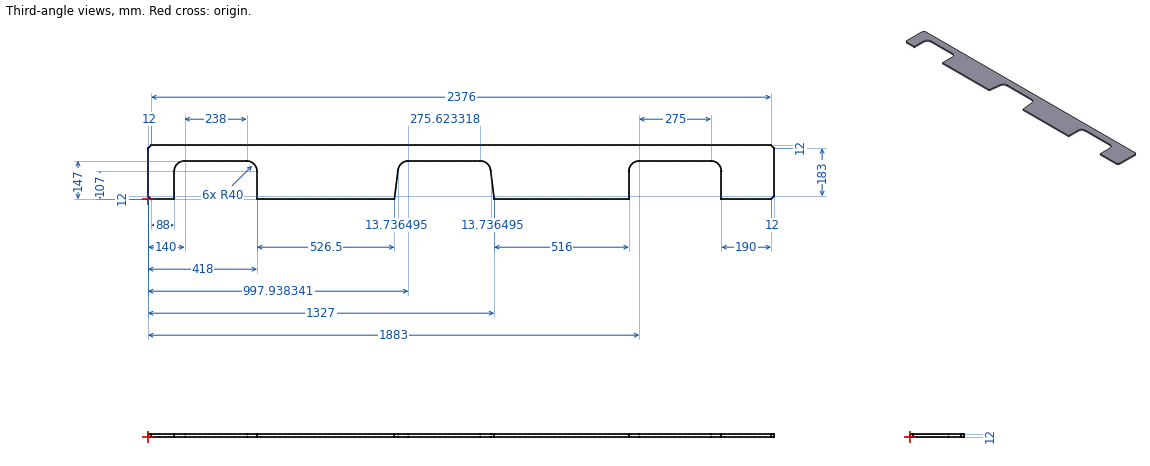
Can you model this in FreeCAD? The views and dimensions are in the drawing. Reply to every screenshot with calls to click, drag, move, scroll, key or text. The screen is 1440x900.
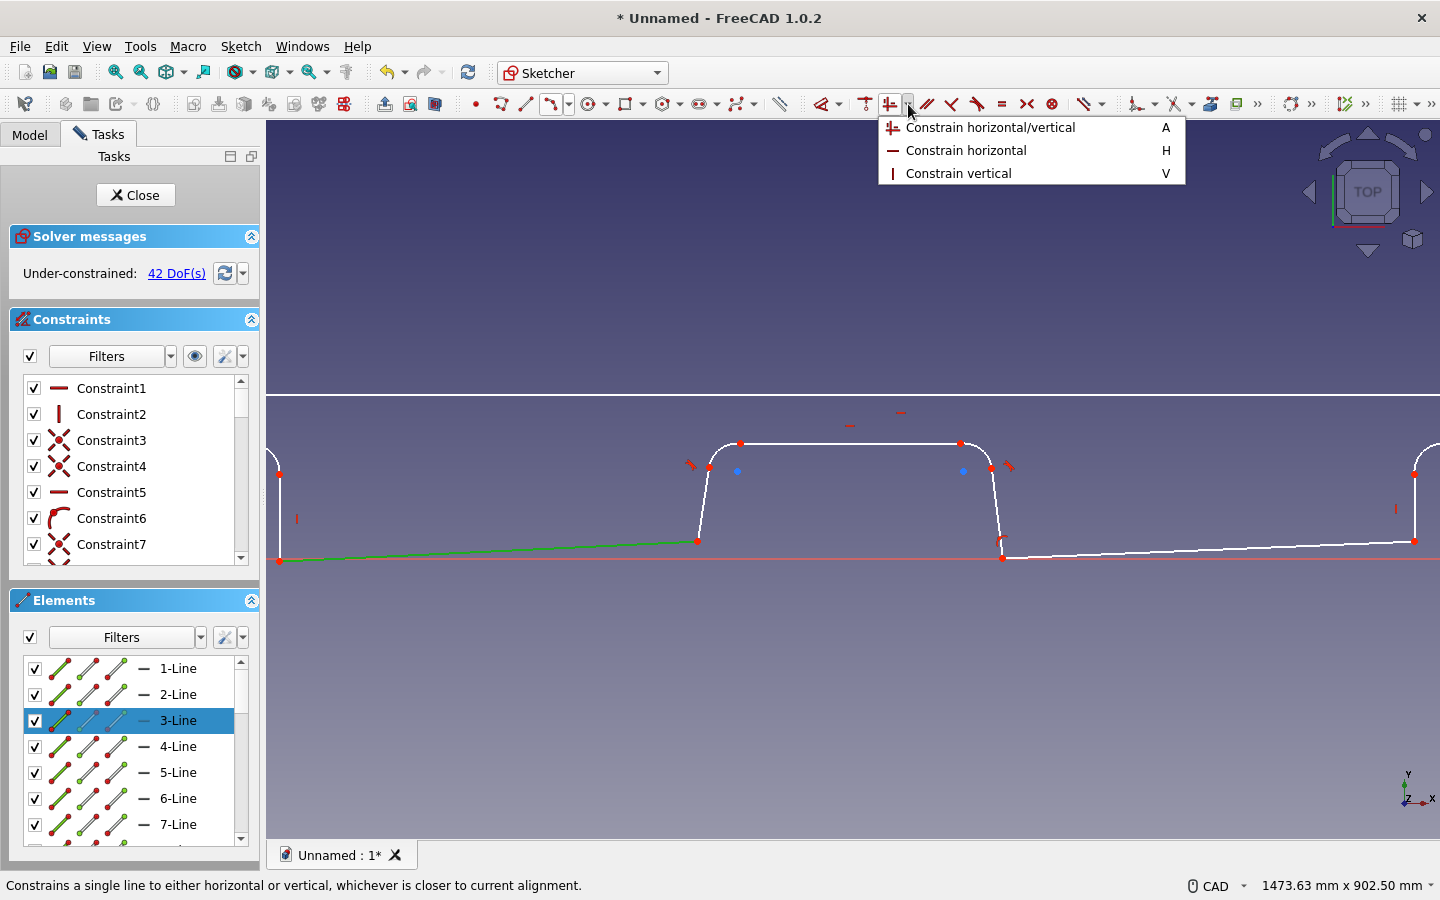
click(1032, 150)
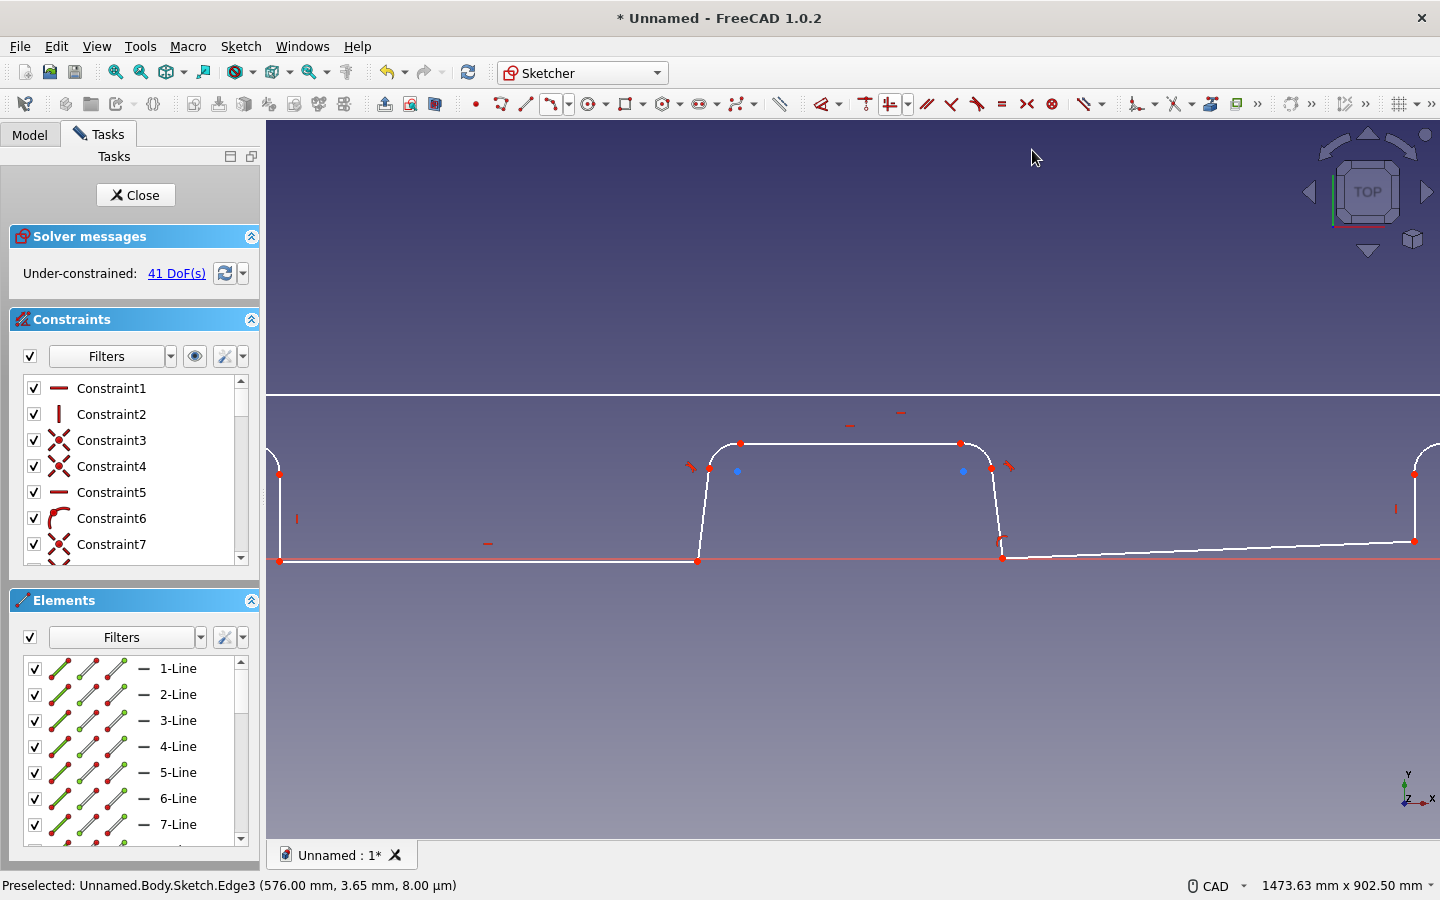
scroll(1250, 548, up, 2)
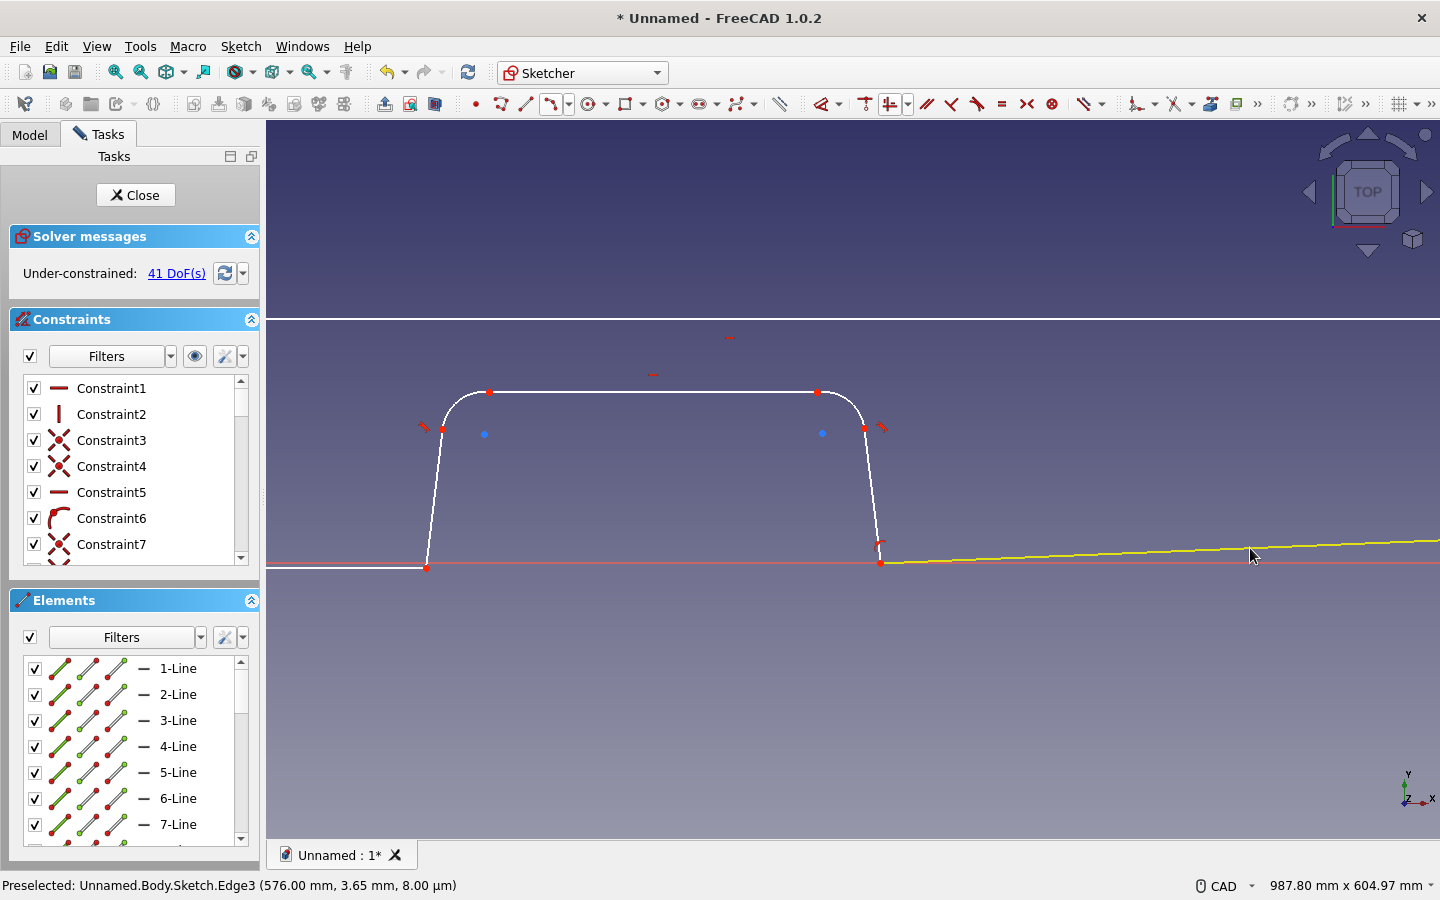
click(1249, 548)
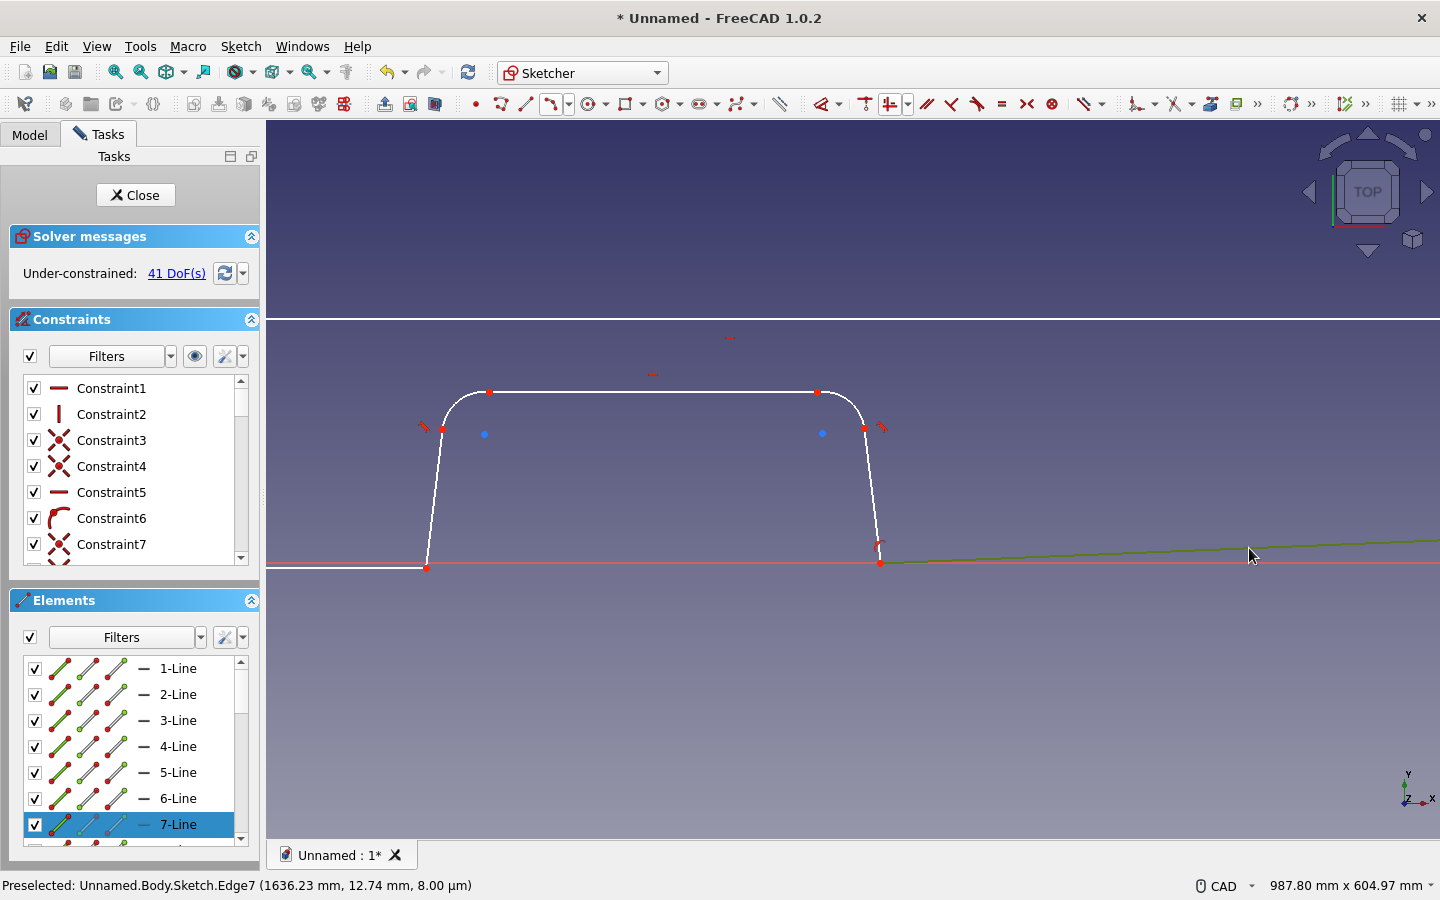
click(908, 104)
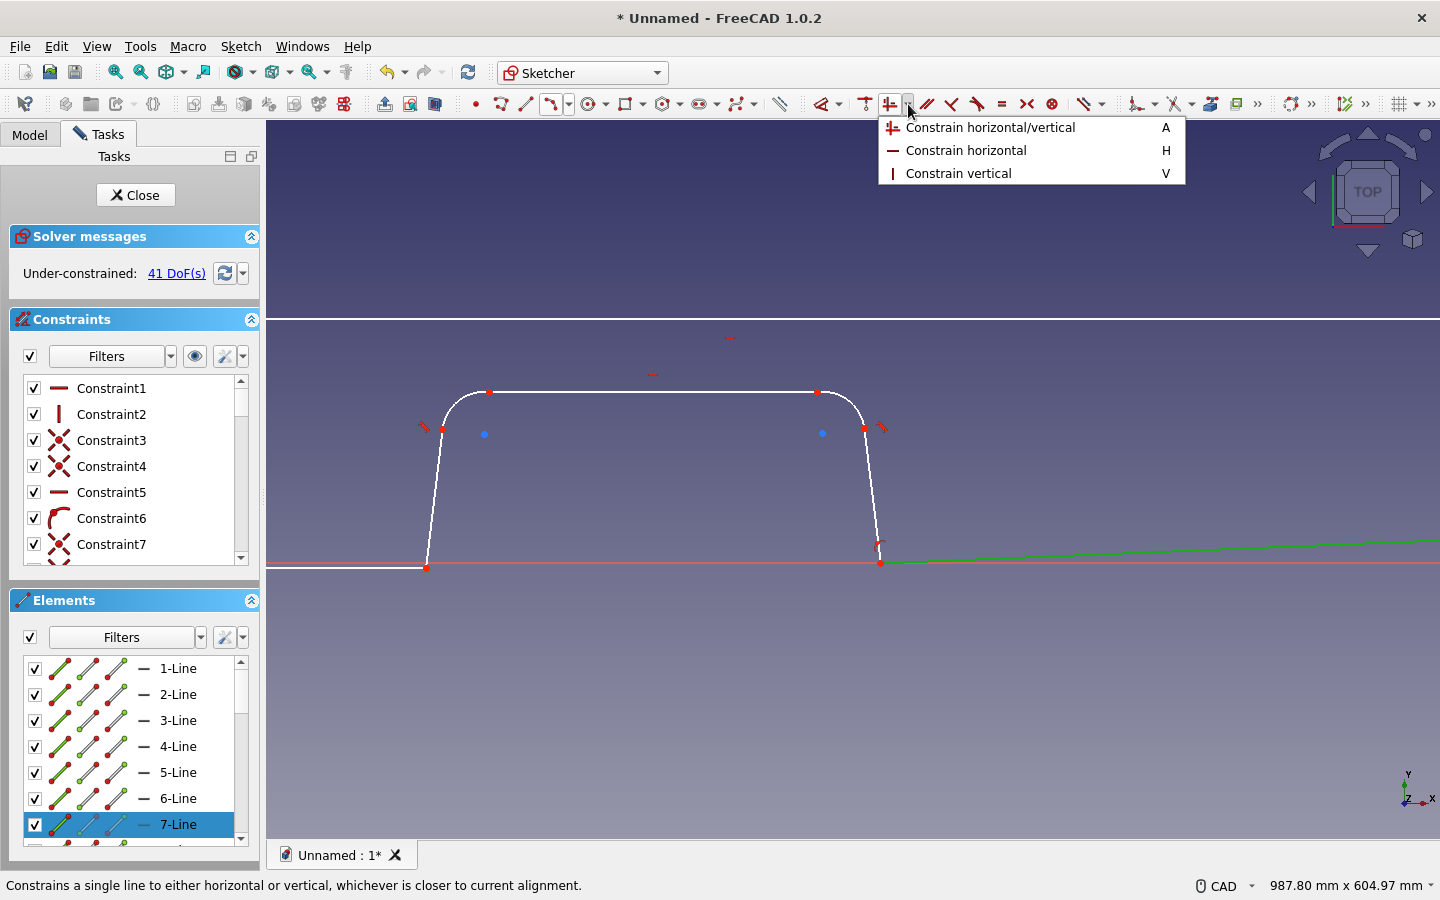
click(1032, 150)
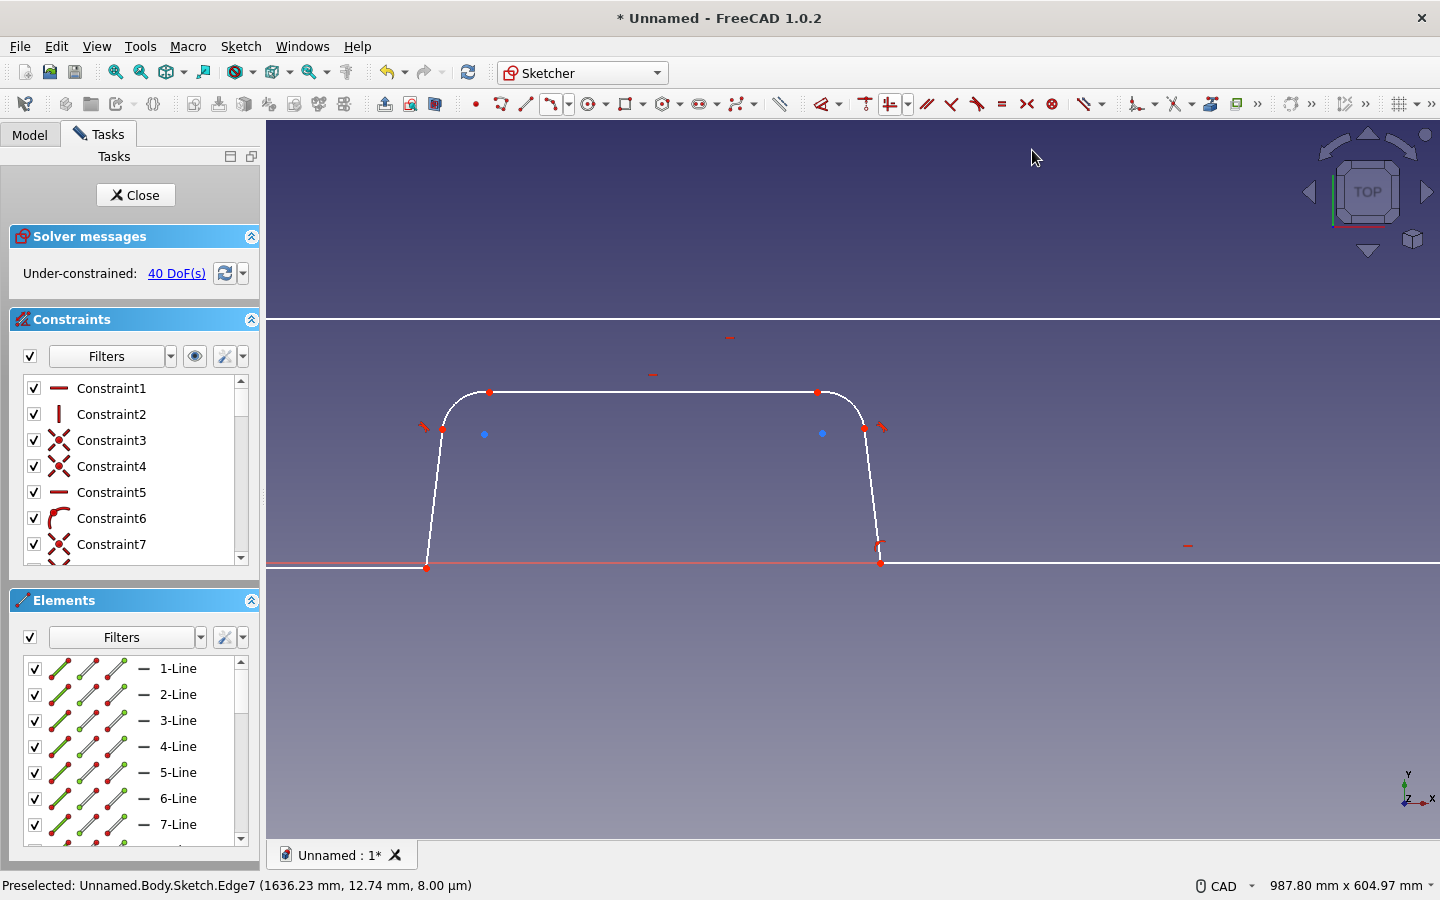
scroll(802, 492, down, 7)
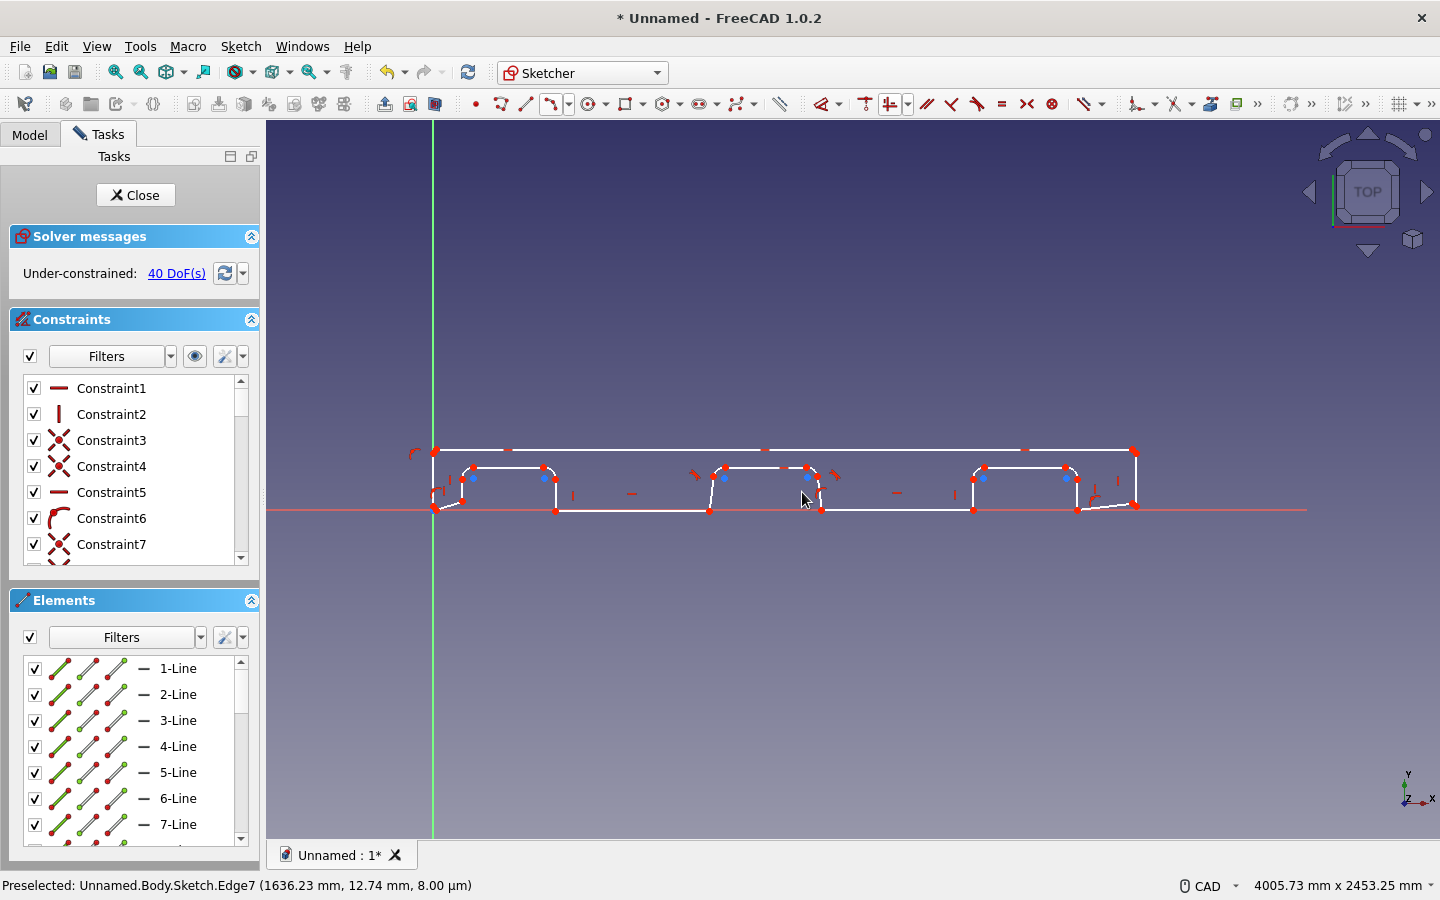
scroll(1116, 506, up, 6)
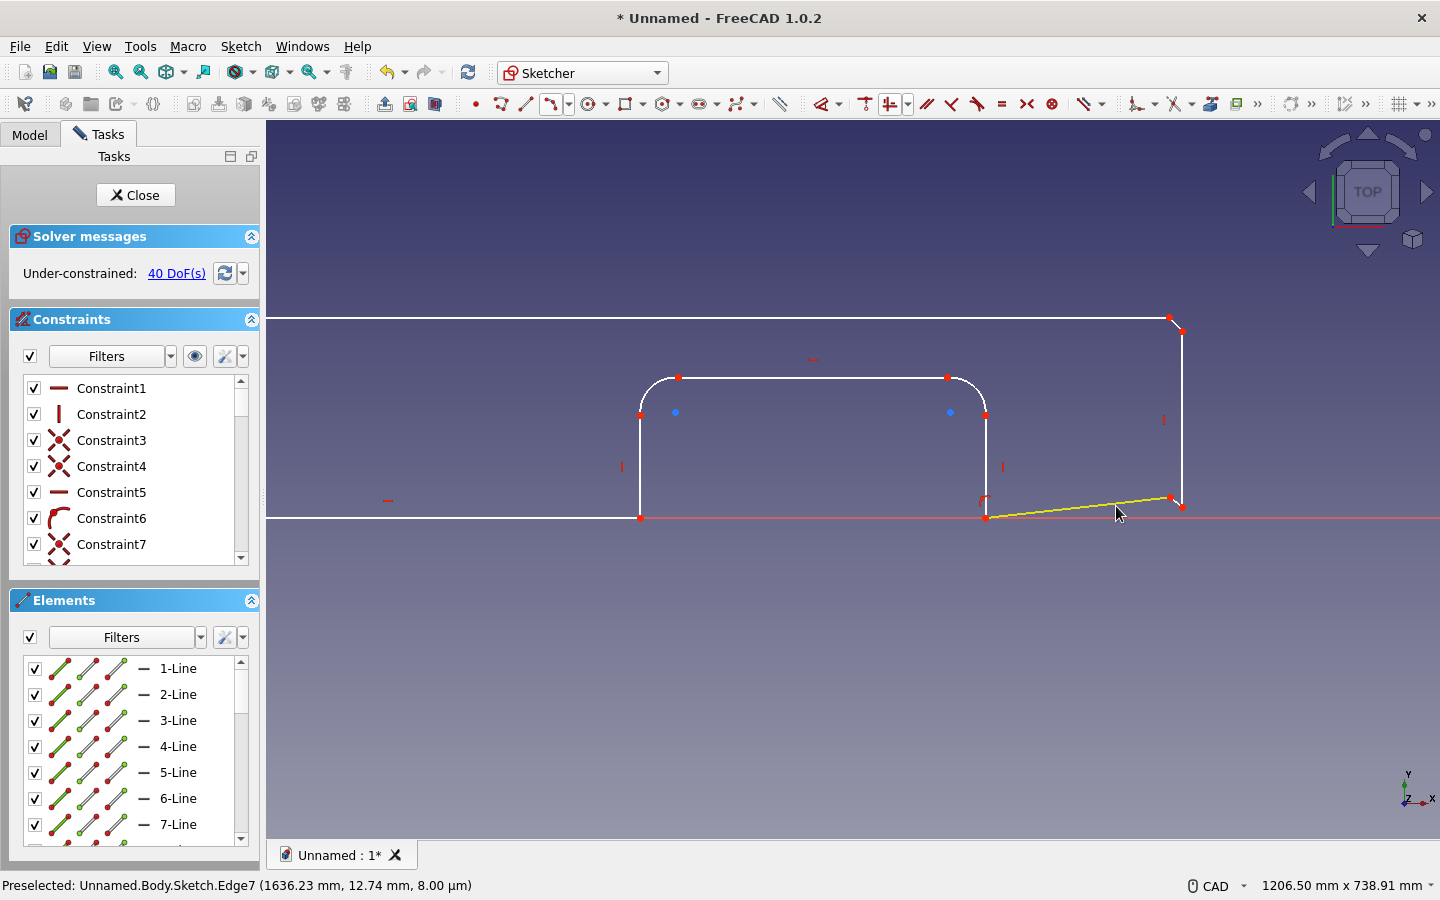
click(1115, 504)